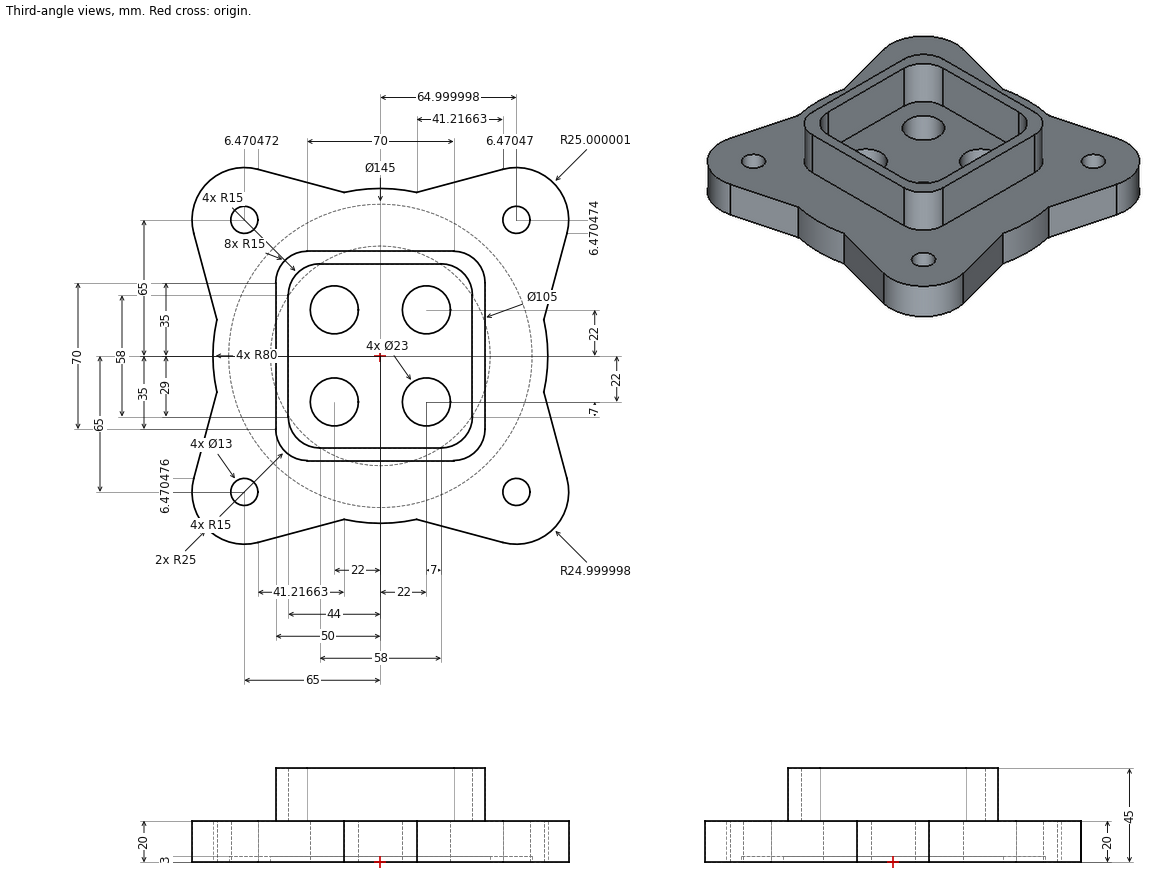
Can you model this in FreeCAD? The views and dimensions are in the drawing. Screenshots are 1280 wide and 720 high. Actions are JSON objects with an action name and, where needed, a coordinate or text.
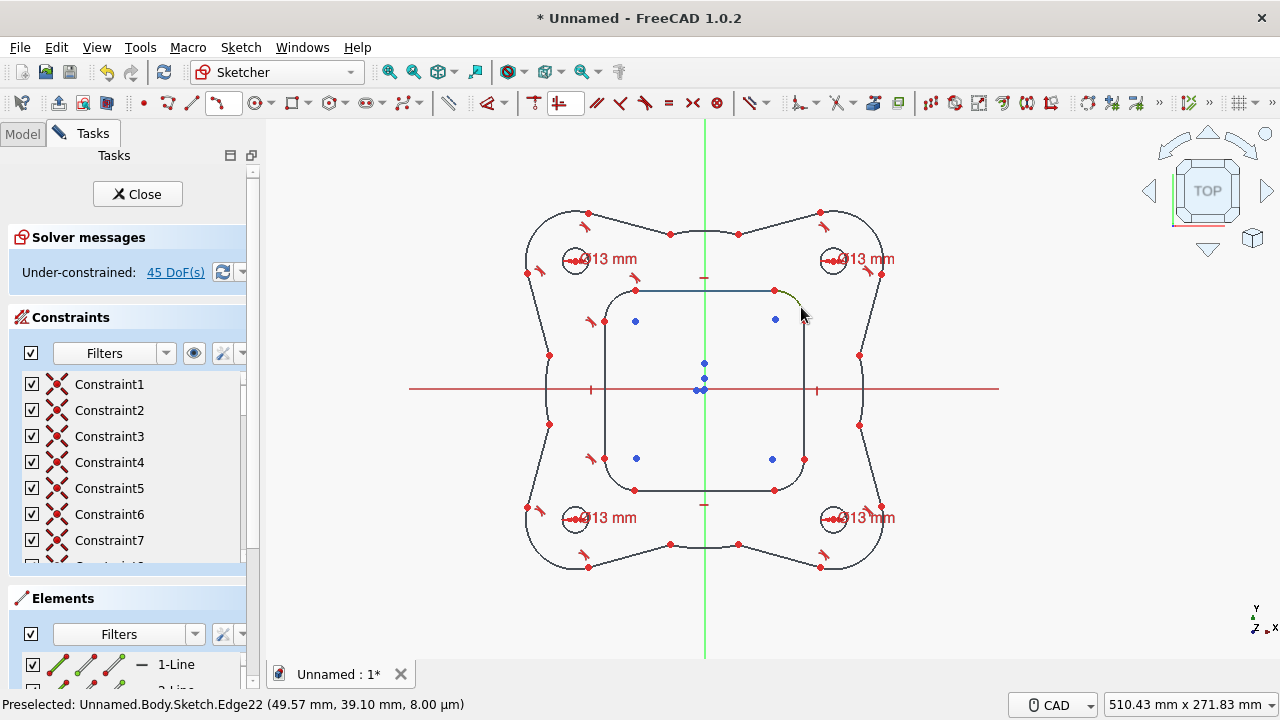
{"action": "key", "text": "t"}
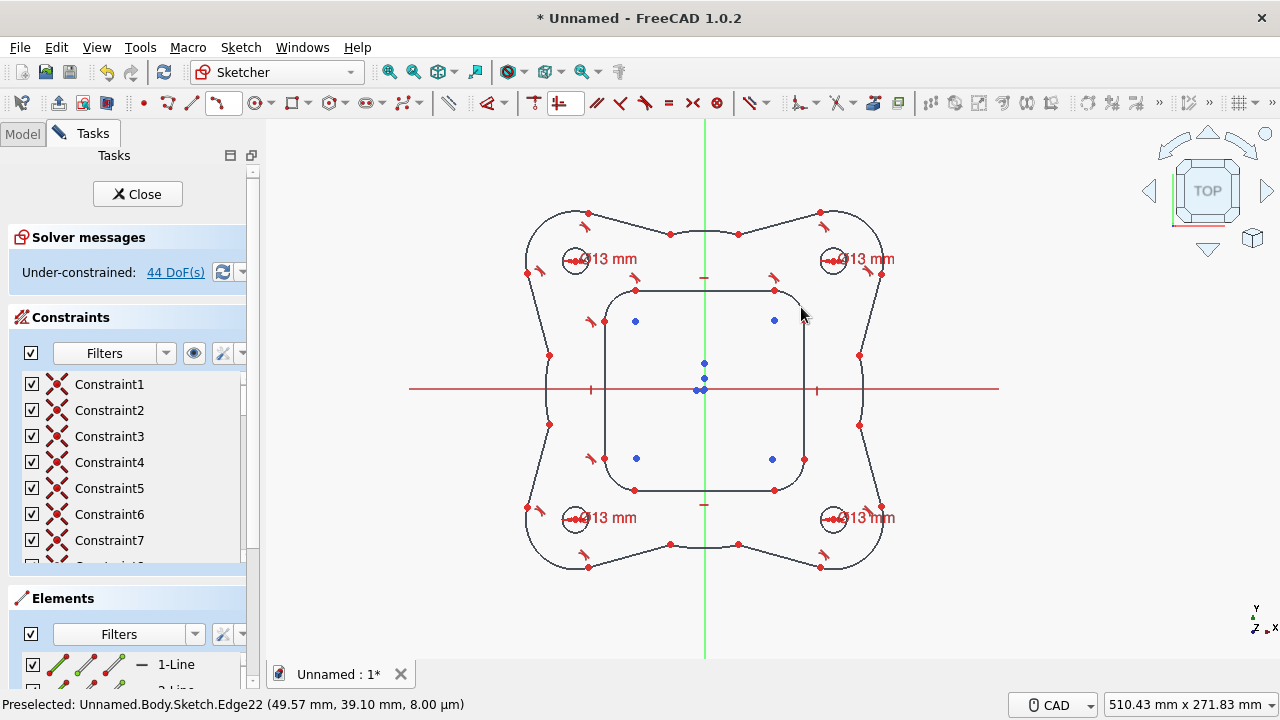
{"action": "left_click", "coordinate": [804, 363]}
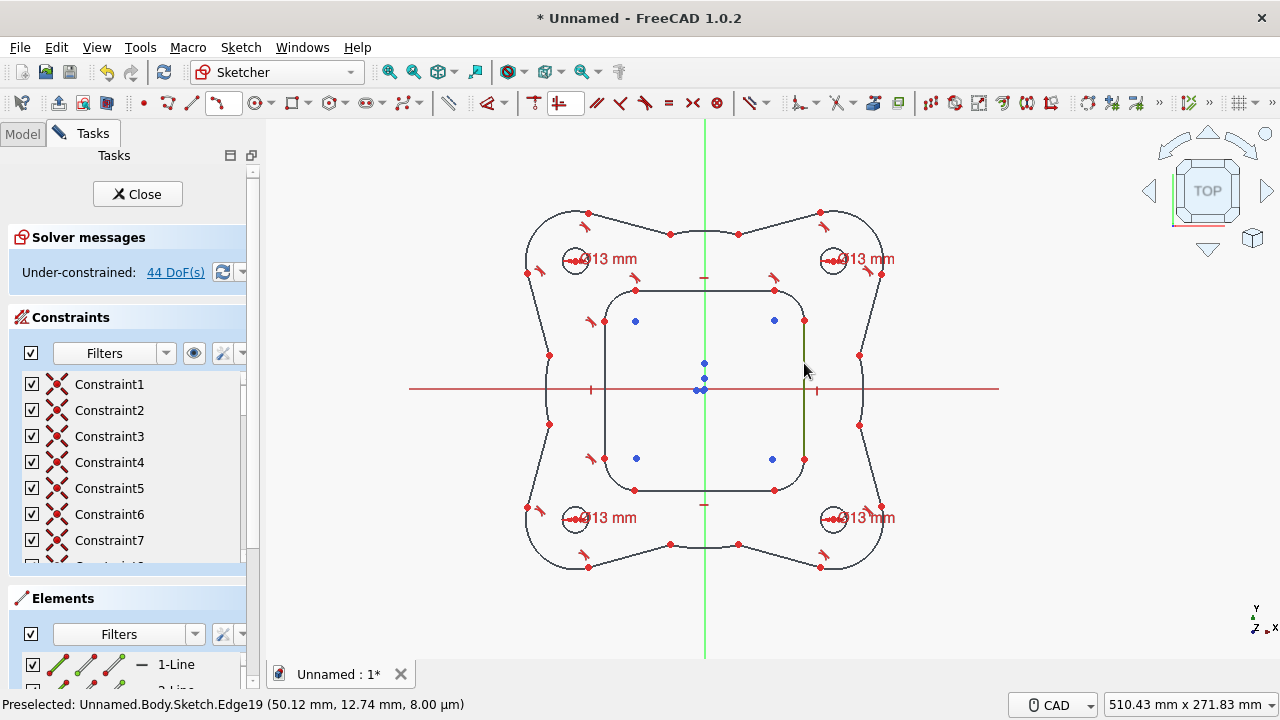
{"action": "left_click", "coordinate": [801, 307]}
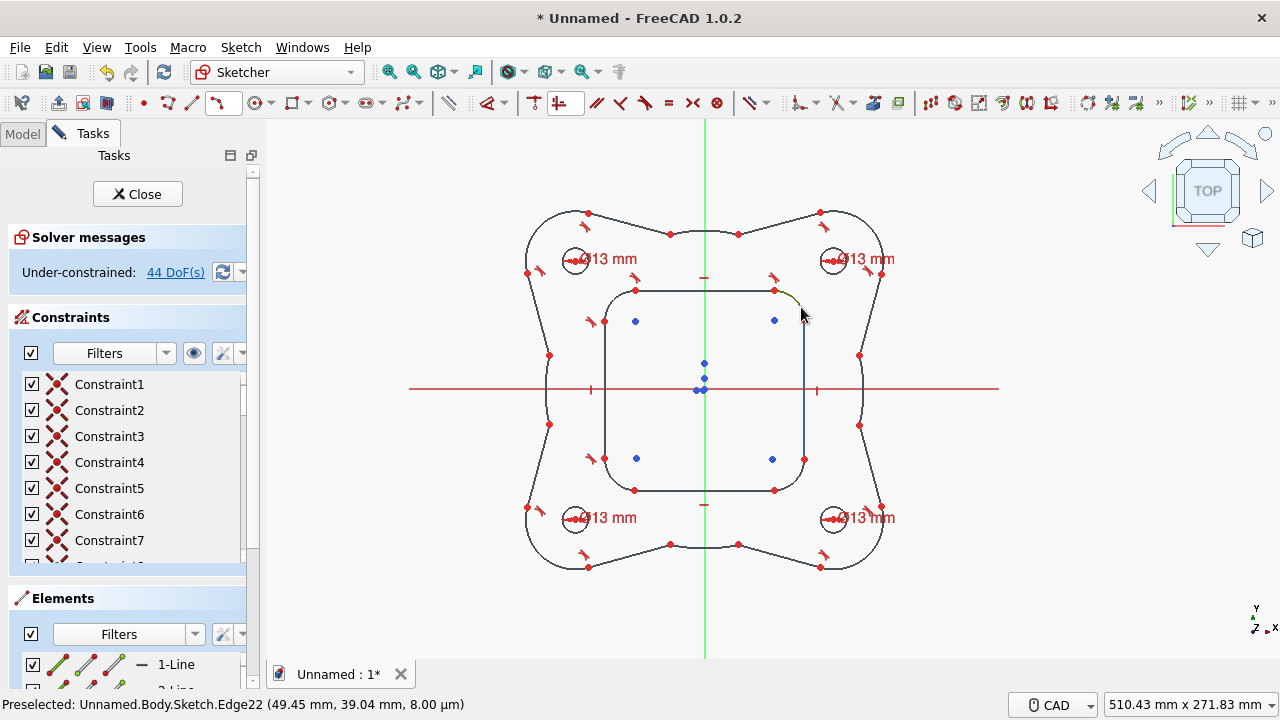
{"action": "key", "text": "t"}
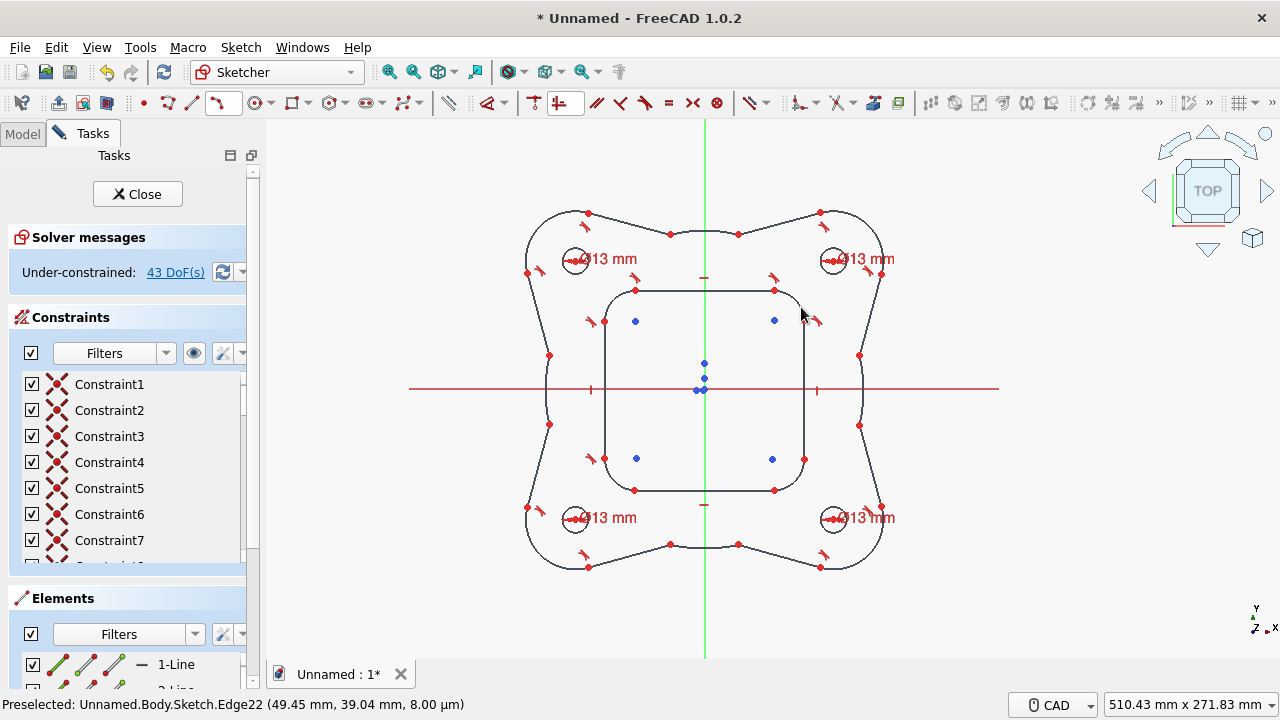
{"action": "left_click", "coordinate": [804, 363]}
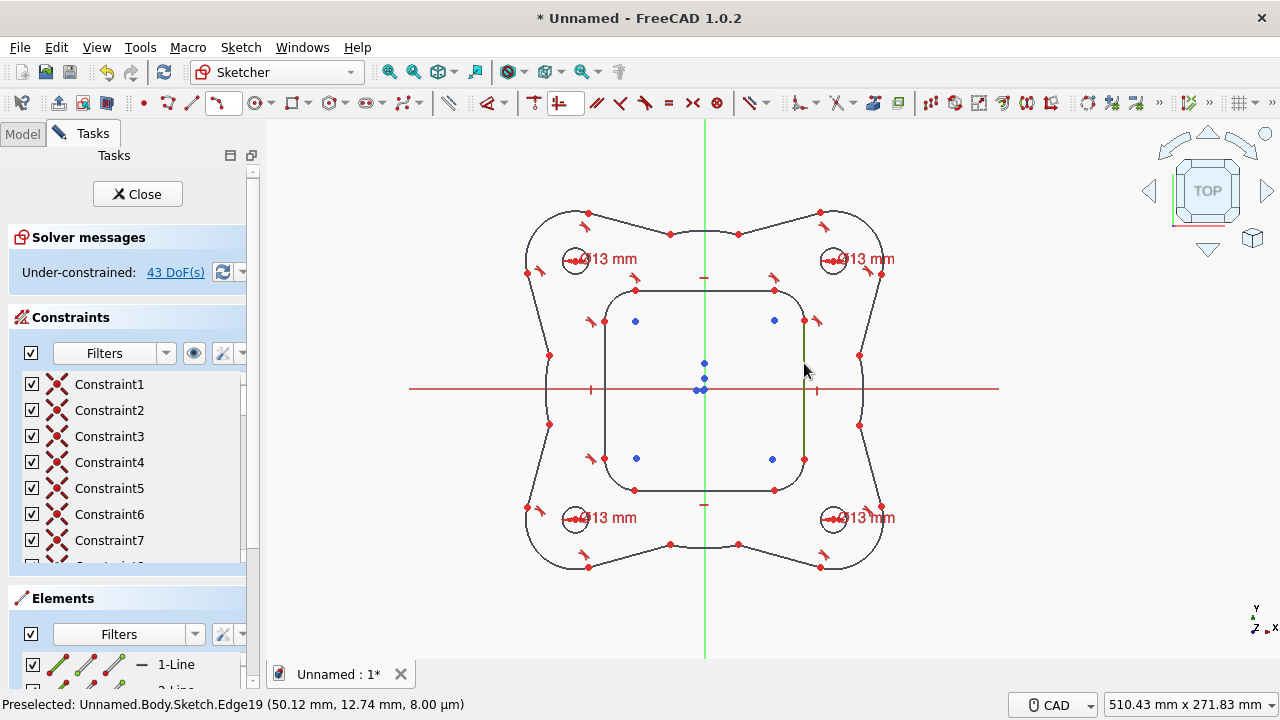
{"action": "left_click", "coordinate": [788, 487]}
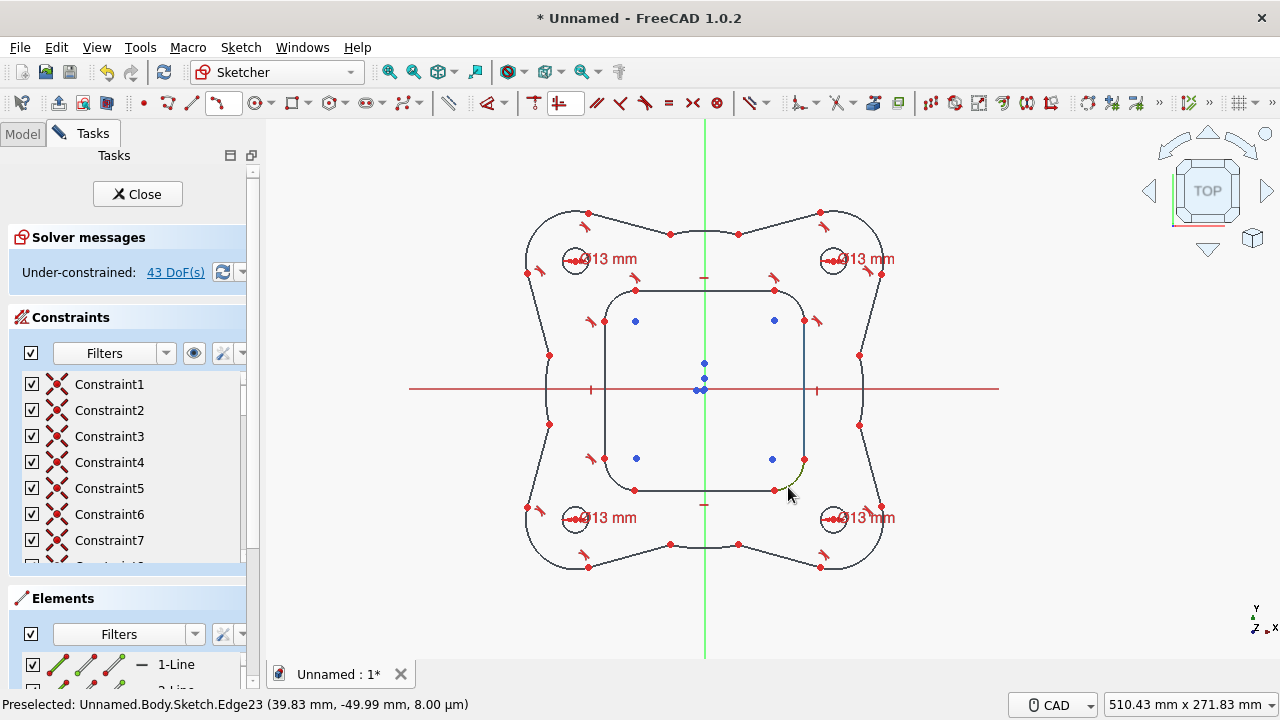
{"action": "left_click", "coordinate": [646, 104]}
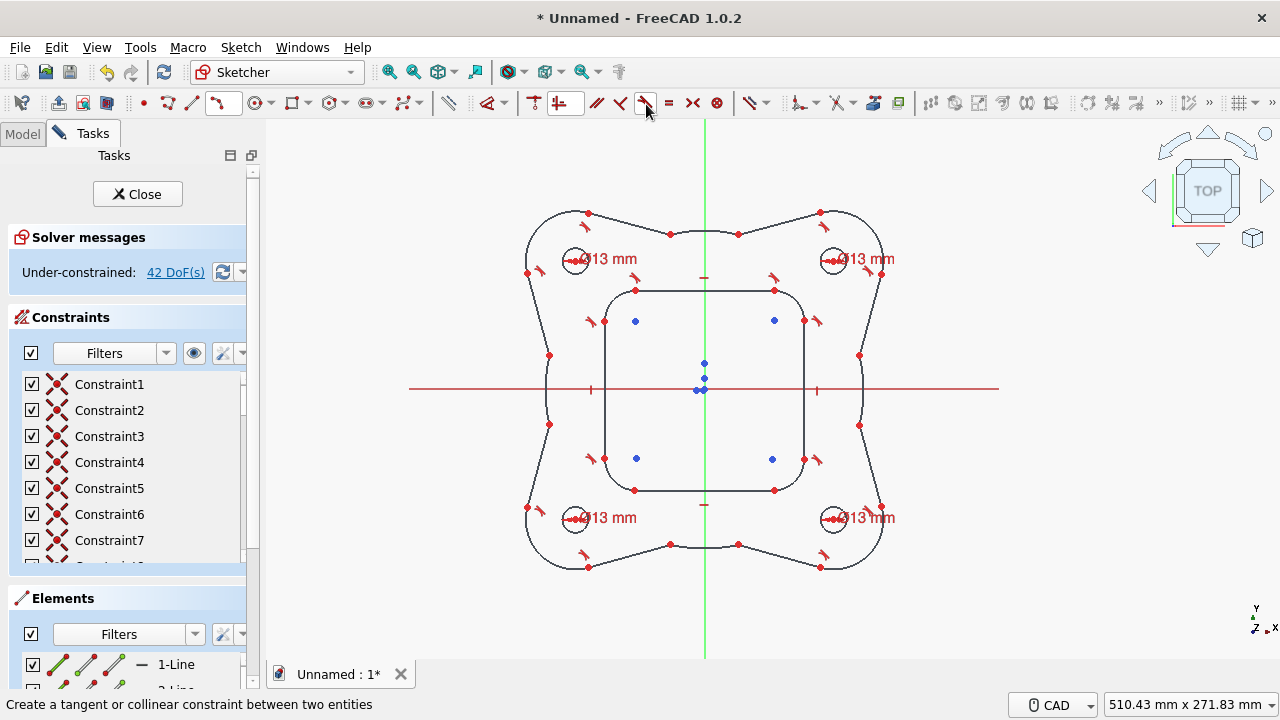
{"action": "left_click", "coordinate": [733, 491]}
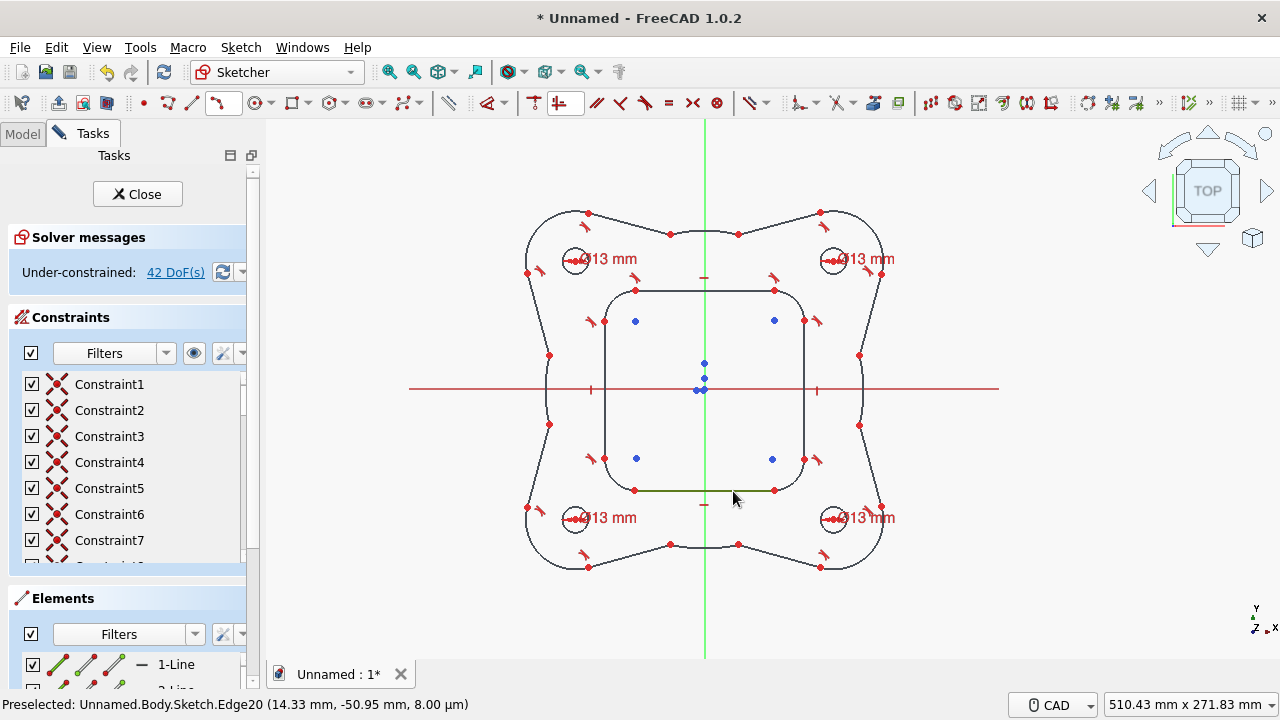
{"action": "left_click", "coordinate": [788, 487]}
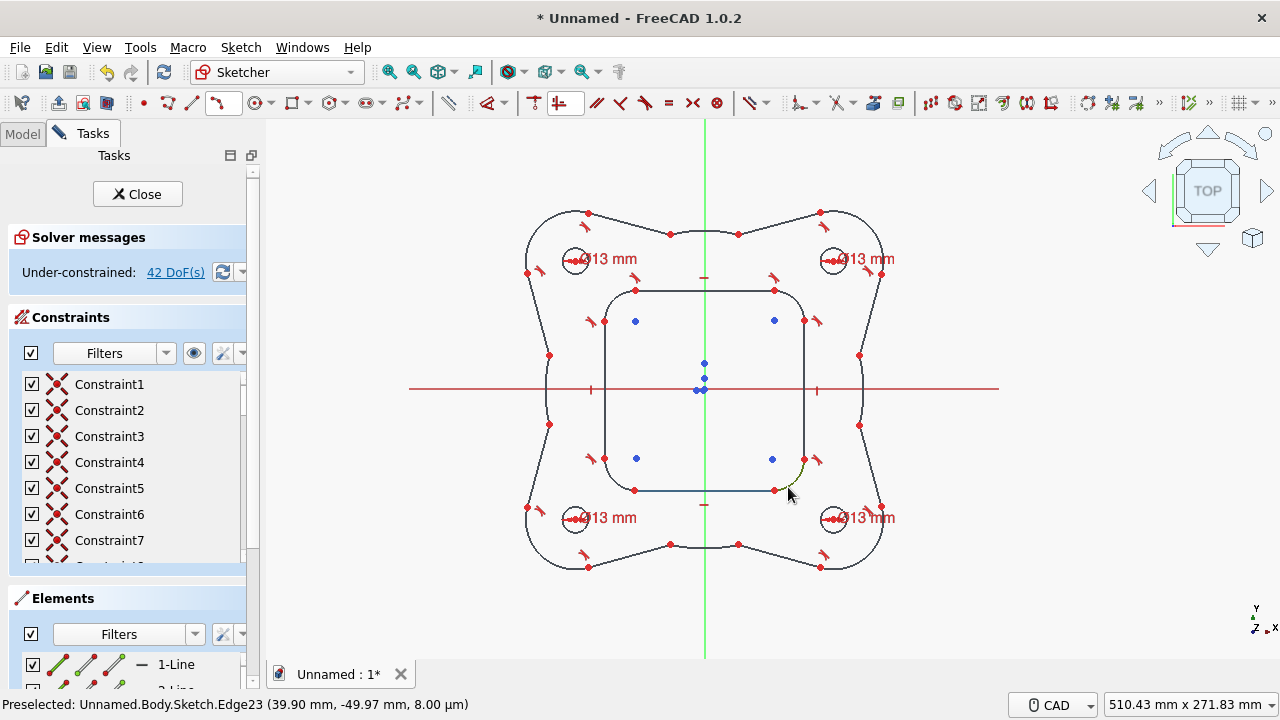
{"action": "left_click", "coordinate": [646, 104]}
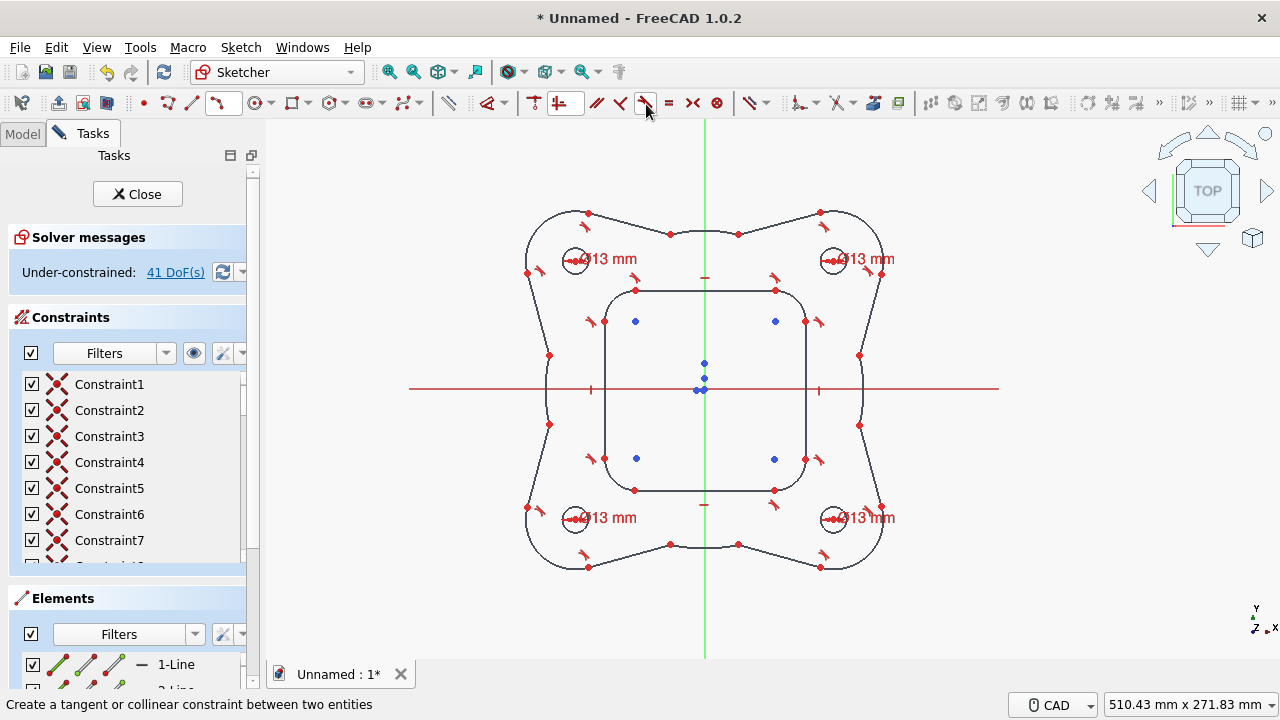
{"action": "left_click", "coordinate": [733, 491]}